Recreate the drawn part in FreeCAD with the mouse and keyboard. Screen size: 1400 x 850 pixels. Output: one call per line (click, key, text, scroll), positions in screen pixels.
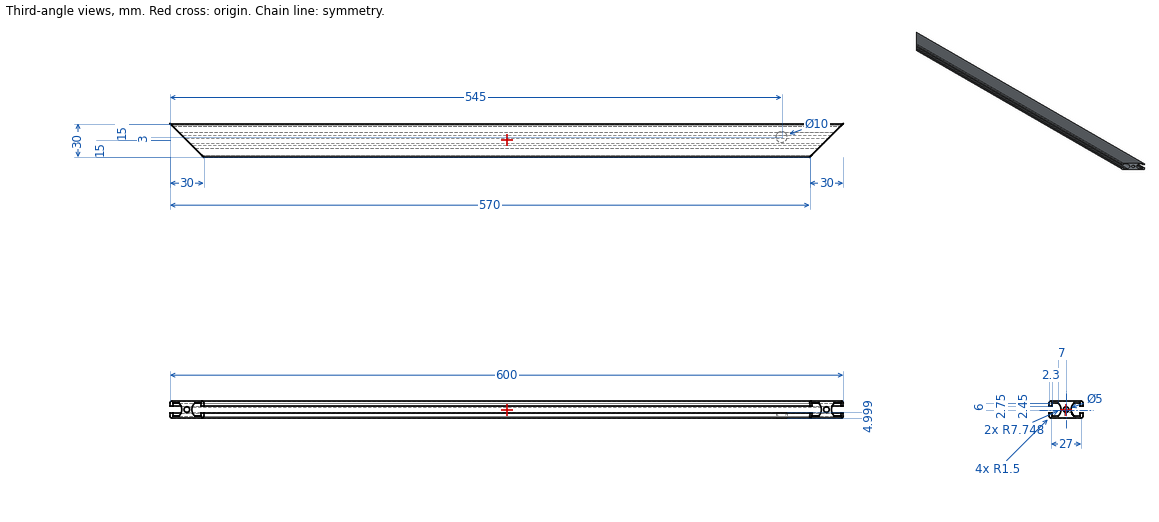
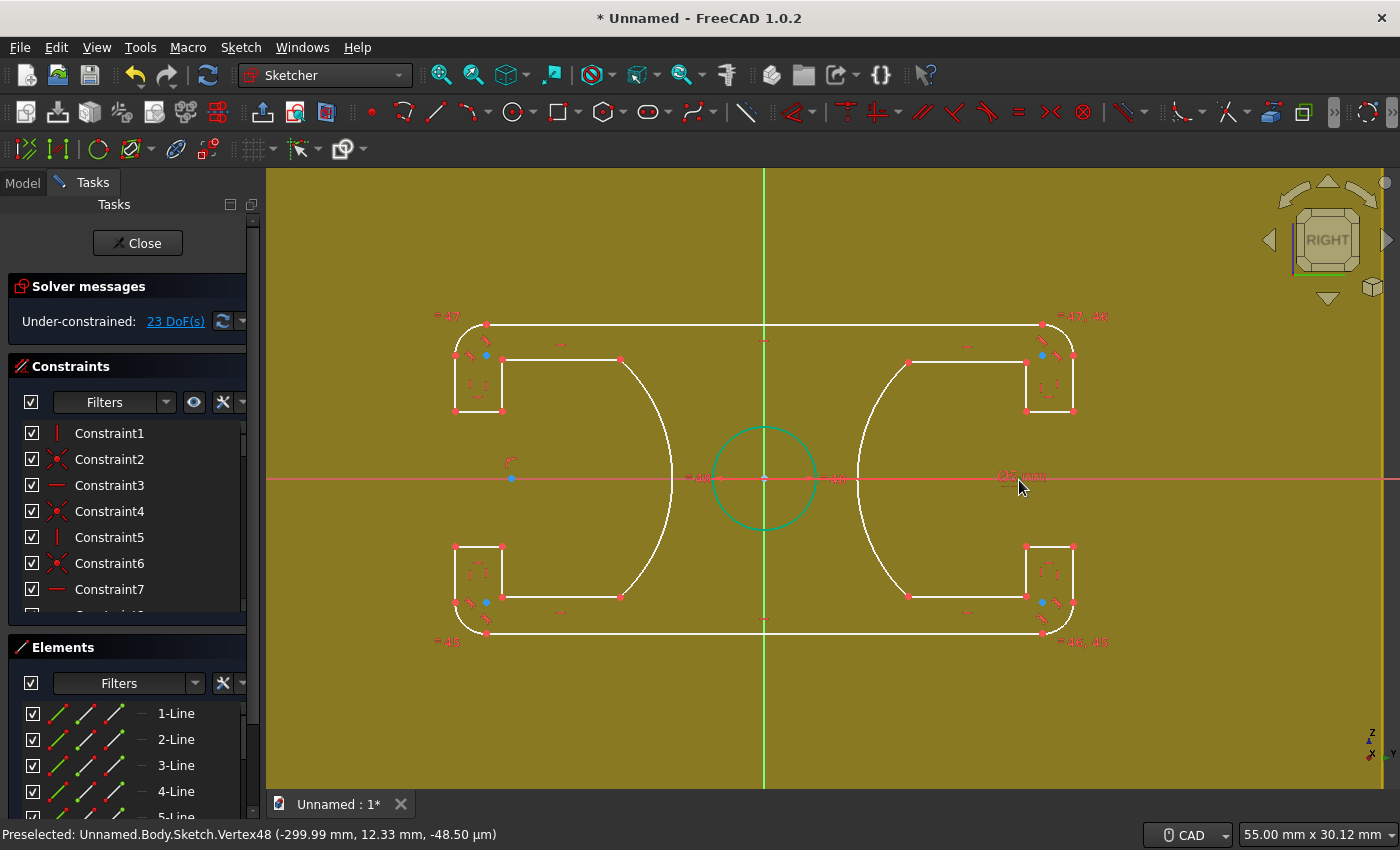
click(361, 478)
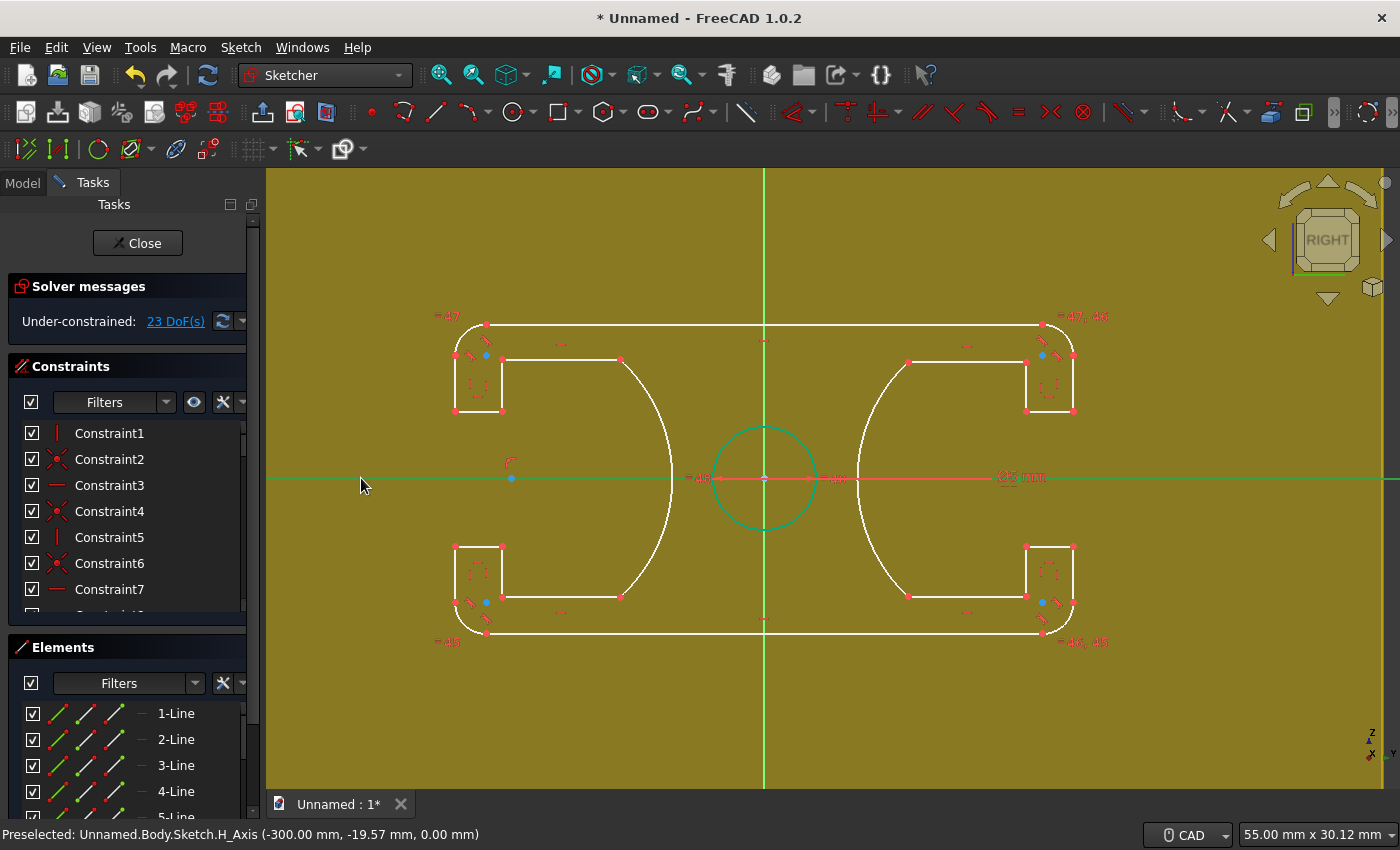
key(c)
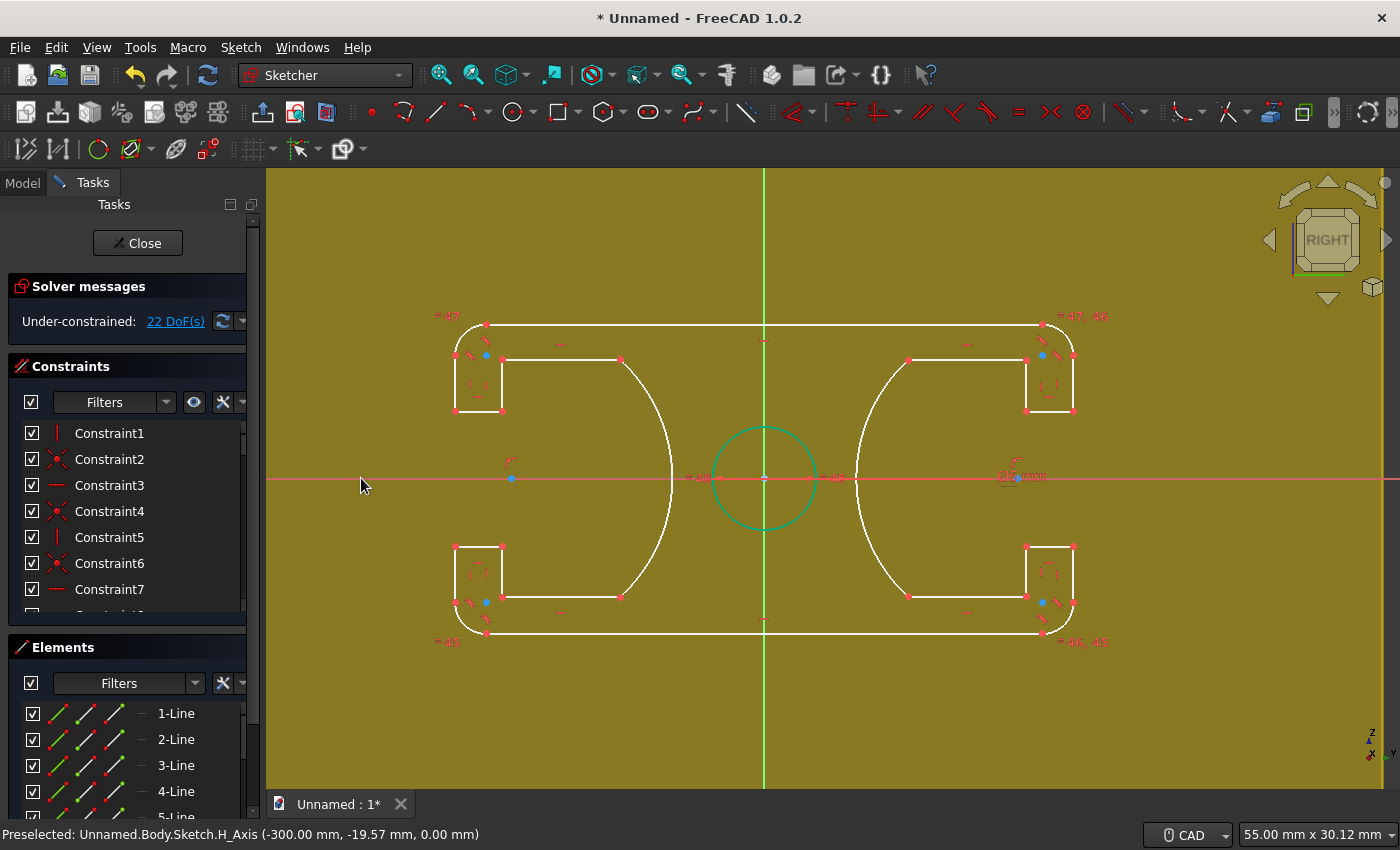
click(1042, 603)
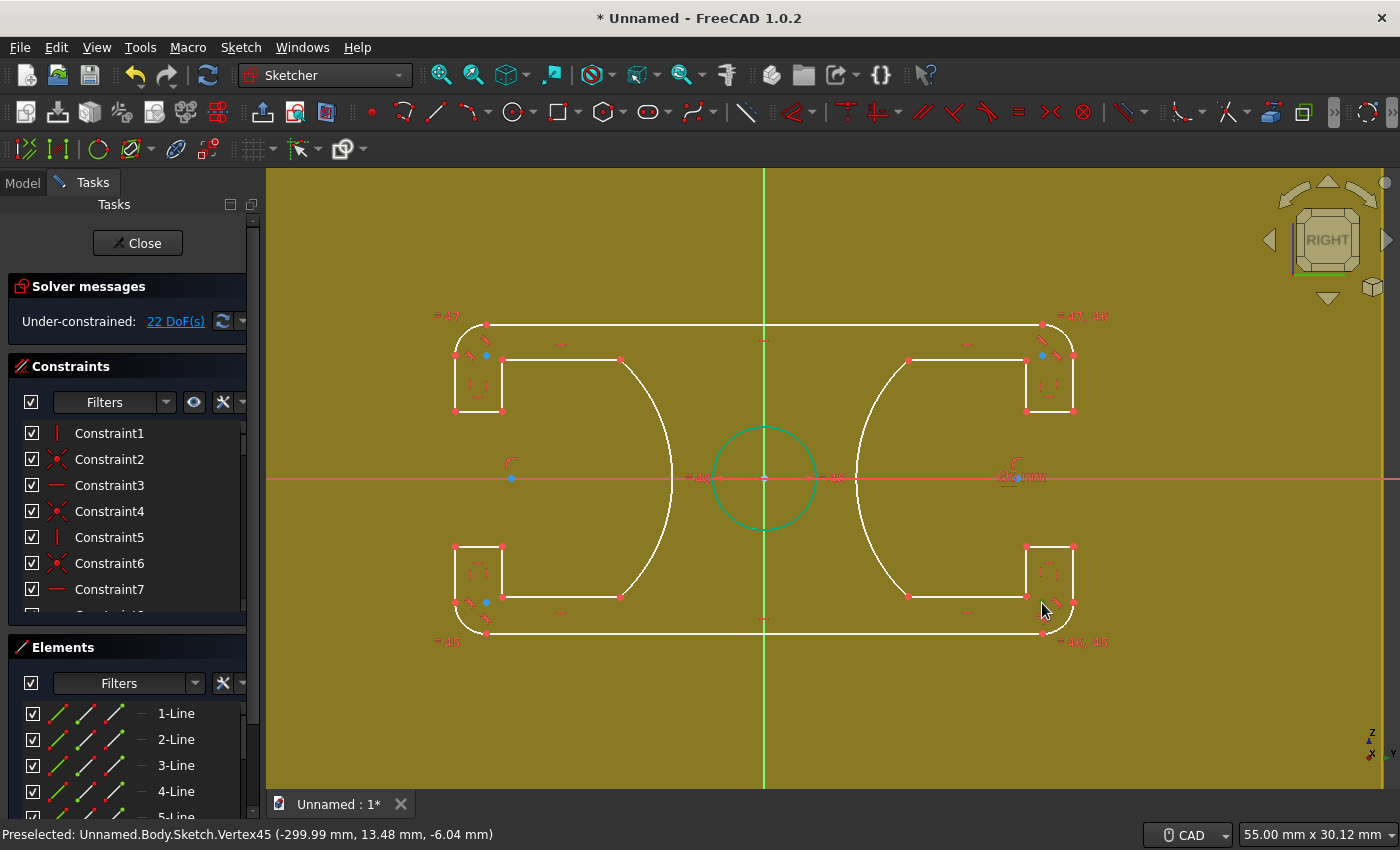
click(1042, 356)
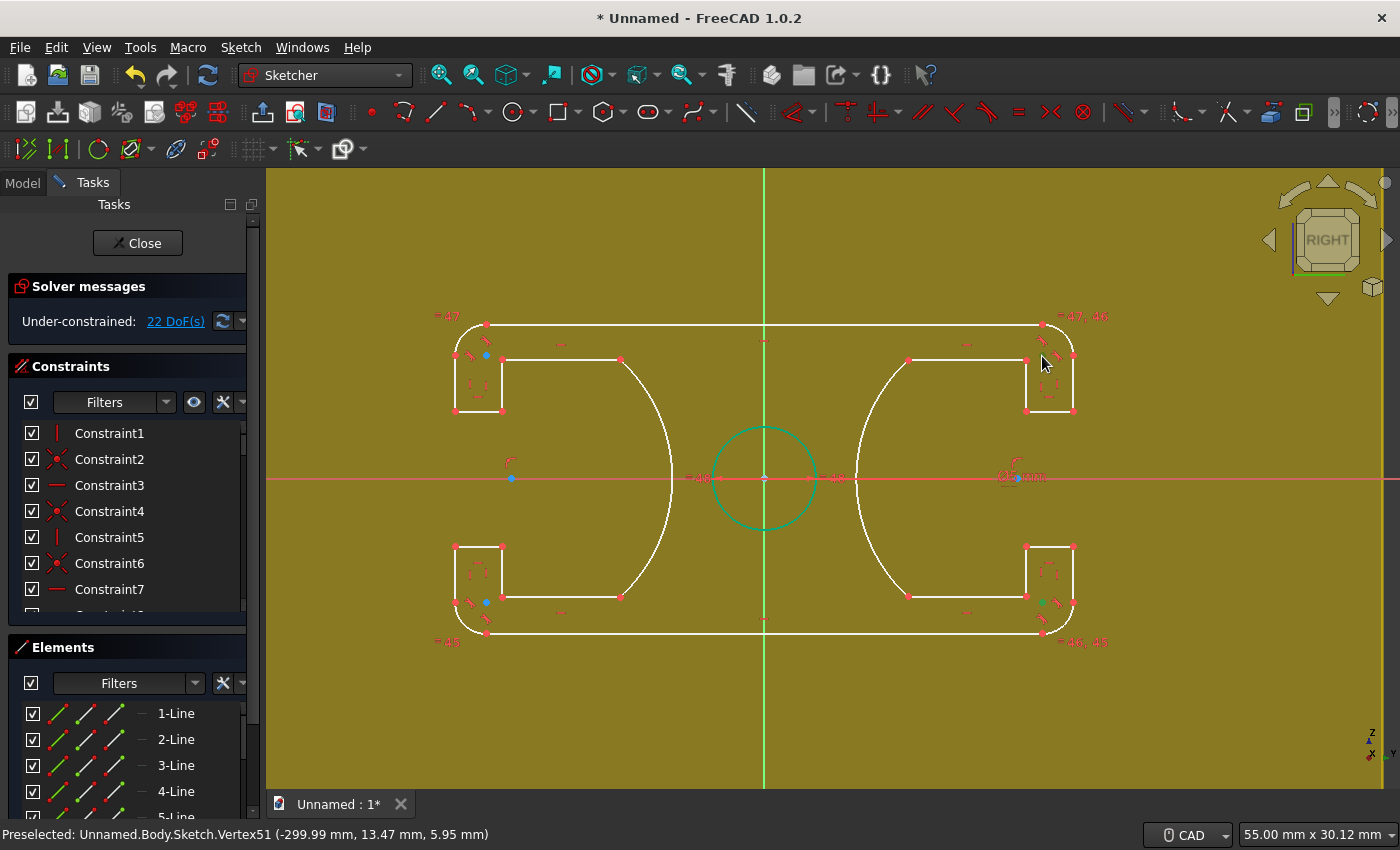
click(361, 478)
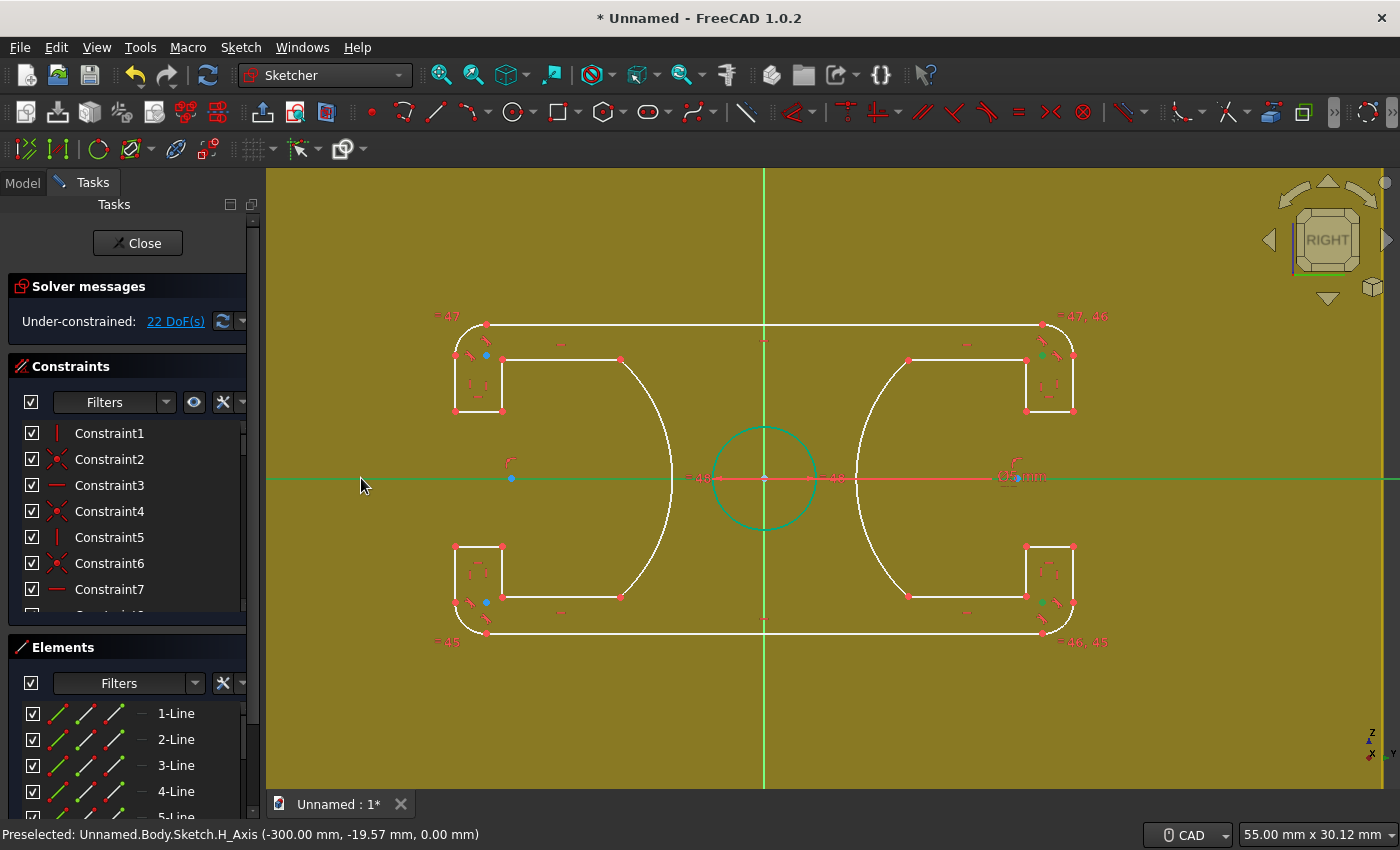
key(s)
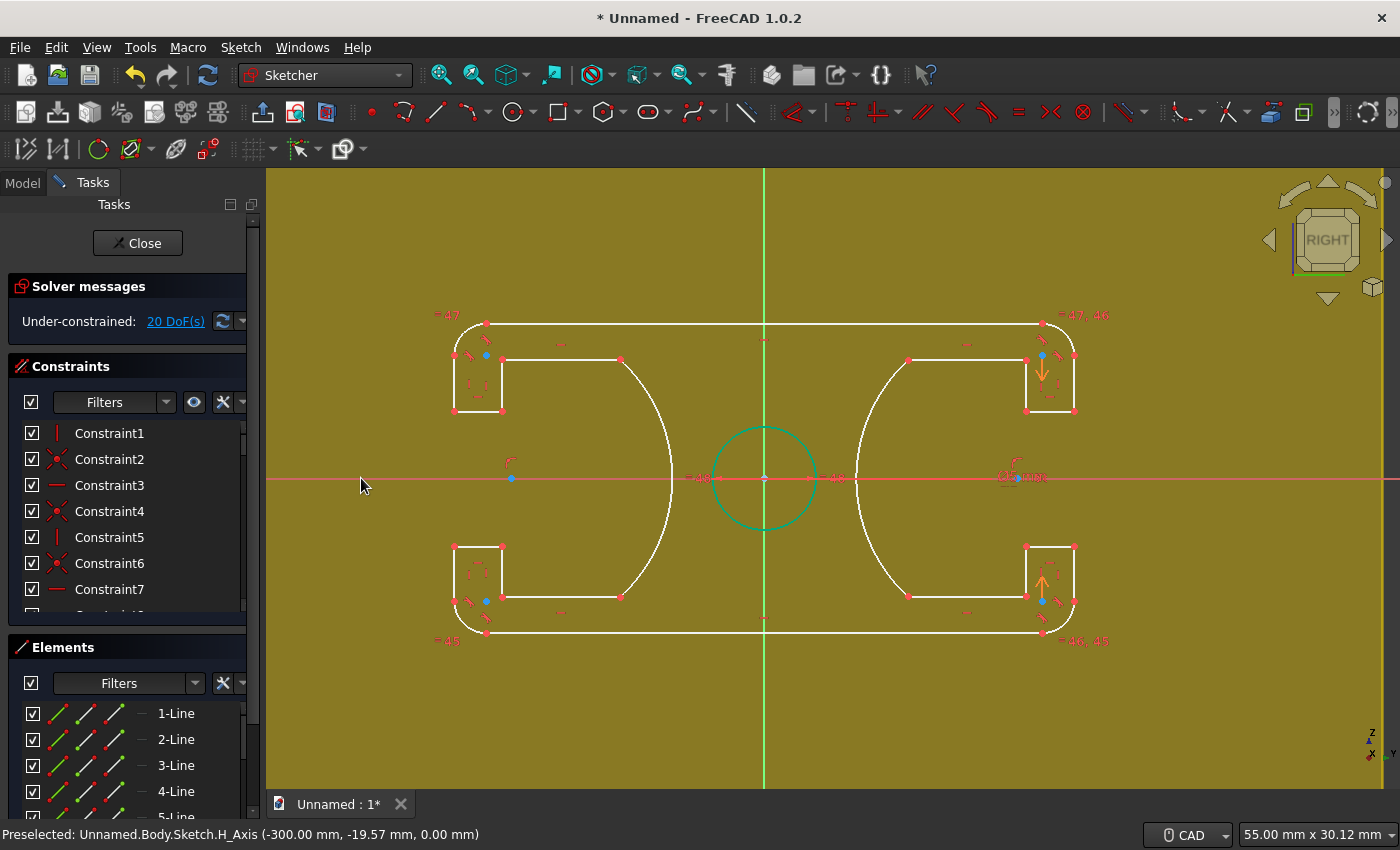
click(502, 360)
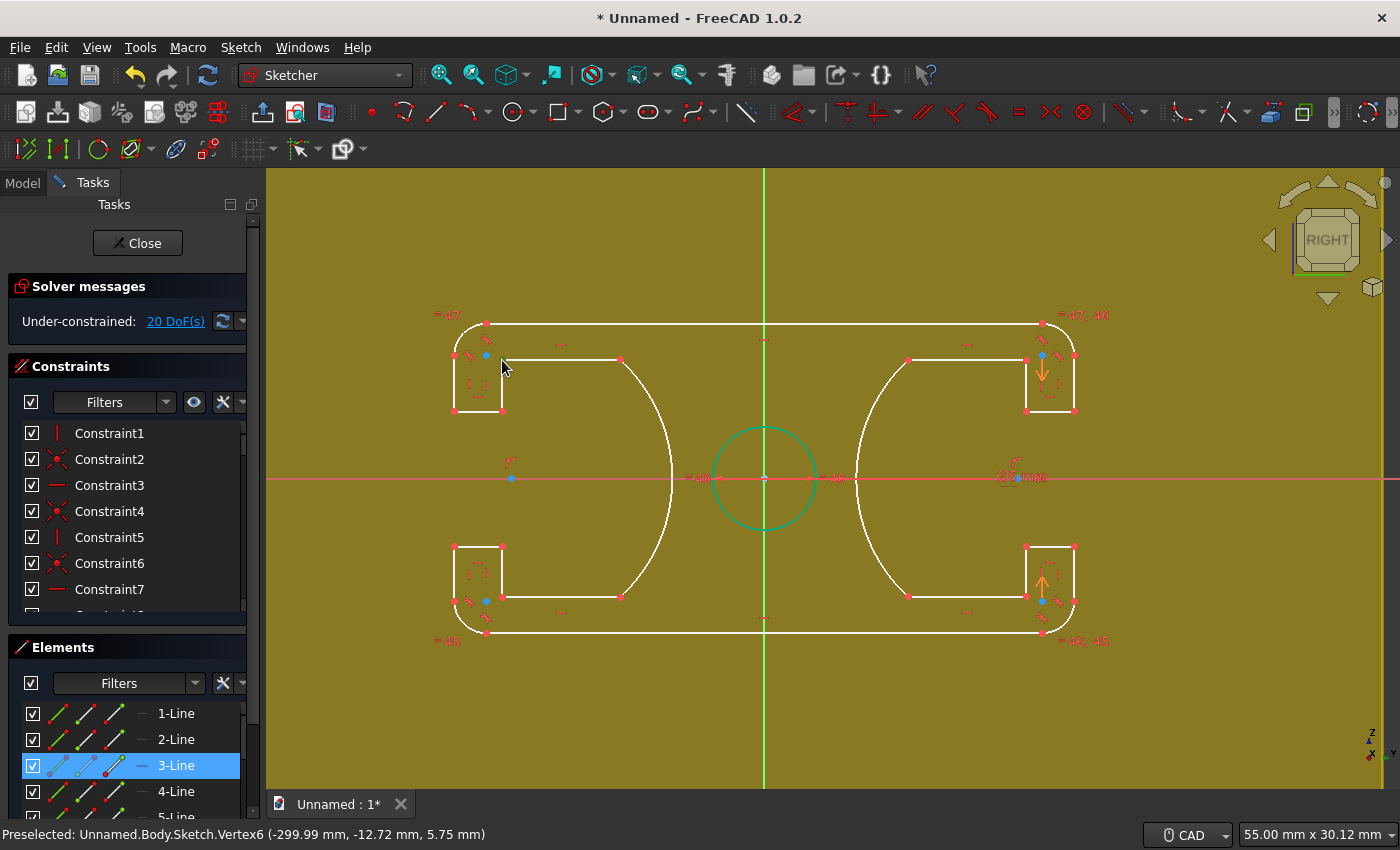
click(502, 597)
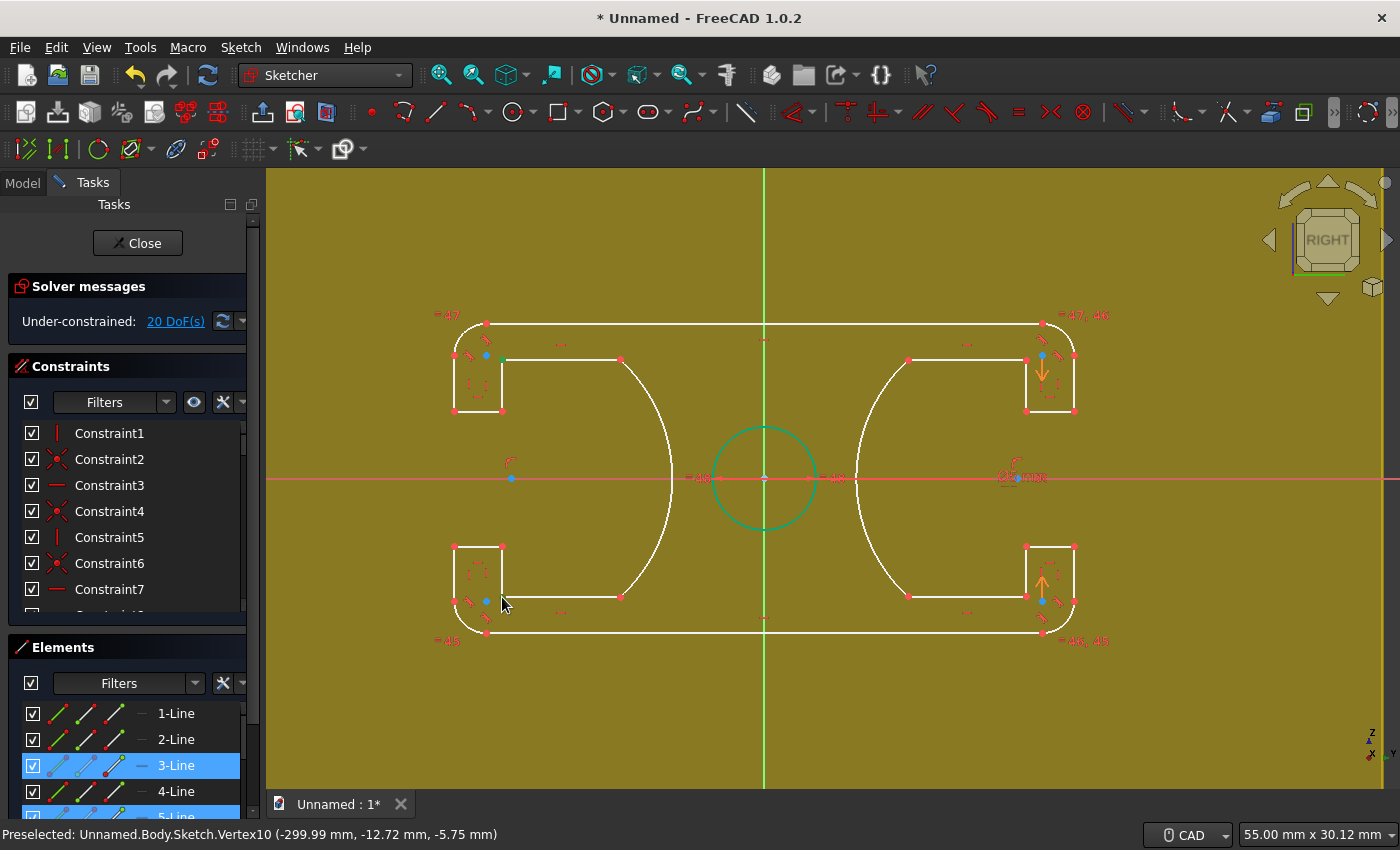
click(361, 478)